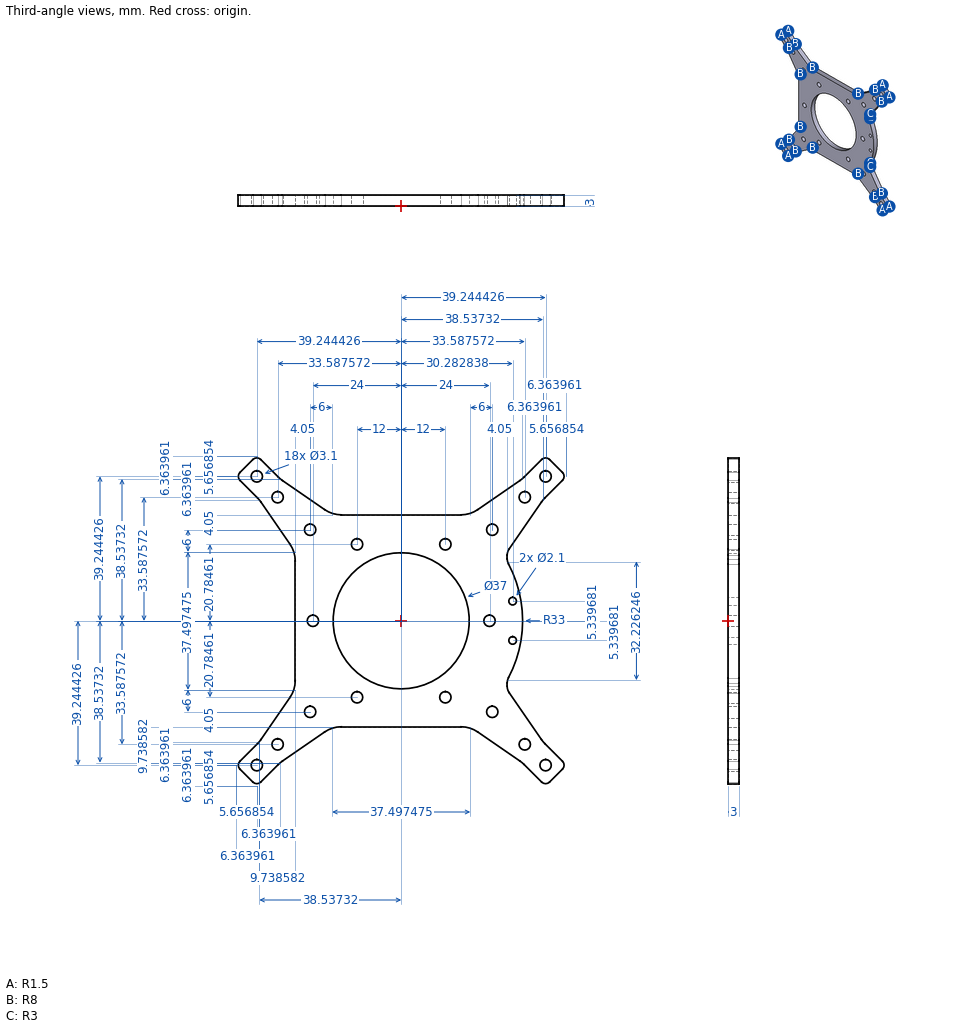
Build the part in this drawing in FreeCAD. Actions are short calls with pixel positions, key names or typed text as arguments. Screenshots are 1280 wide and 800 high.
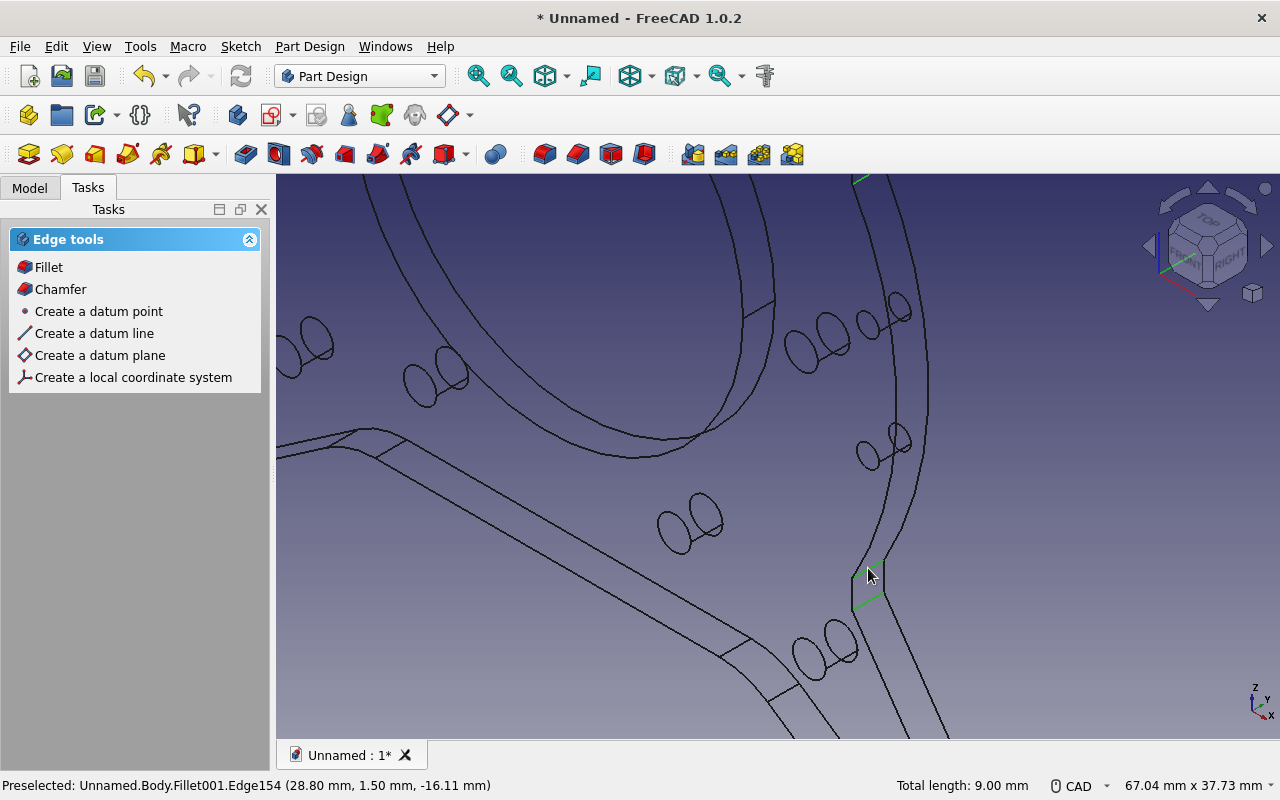
click(479, 76)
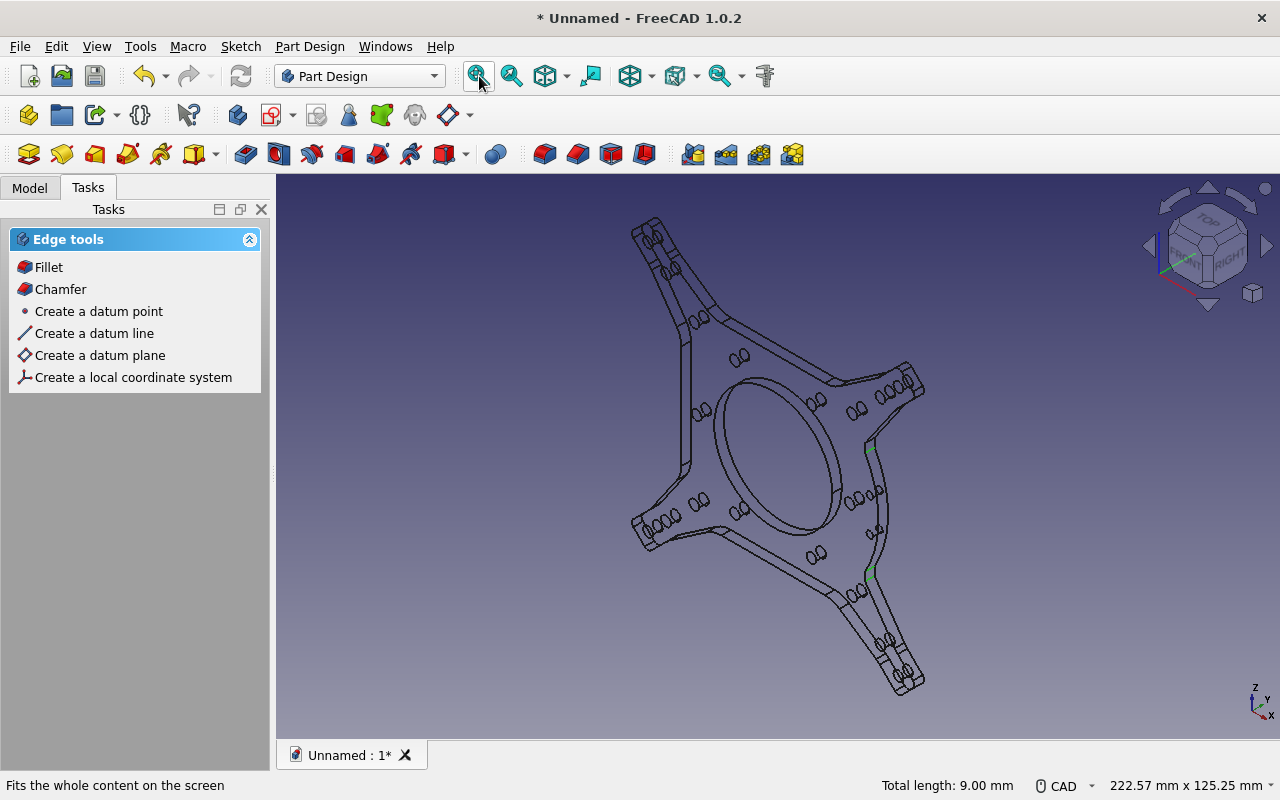
key(2)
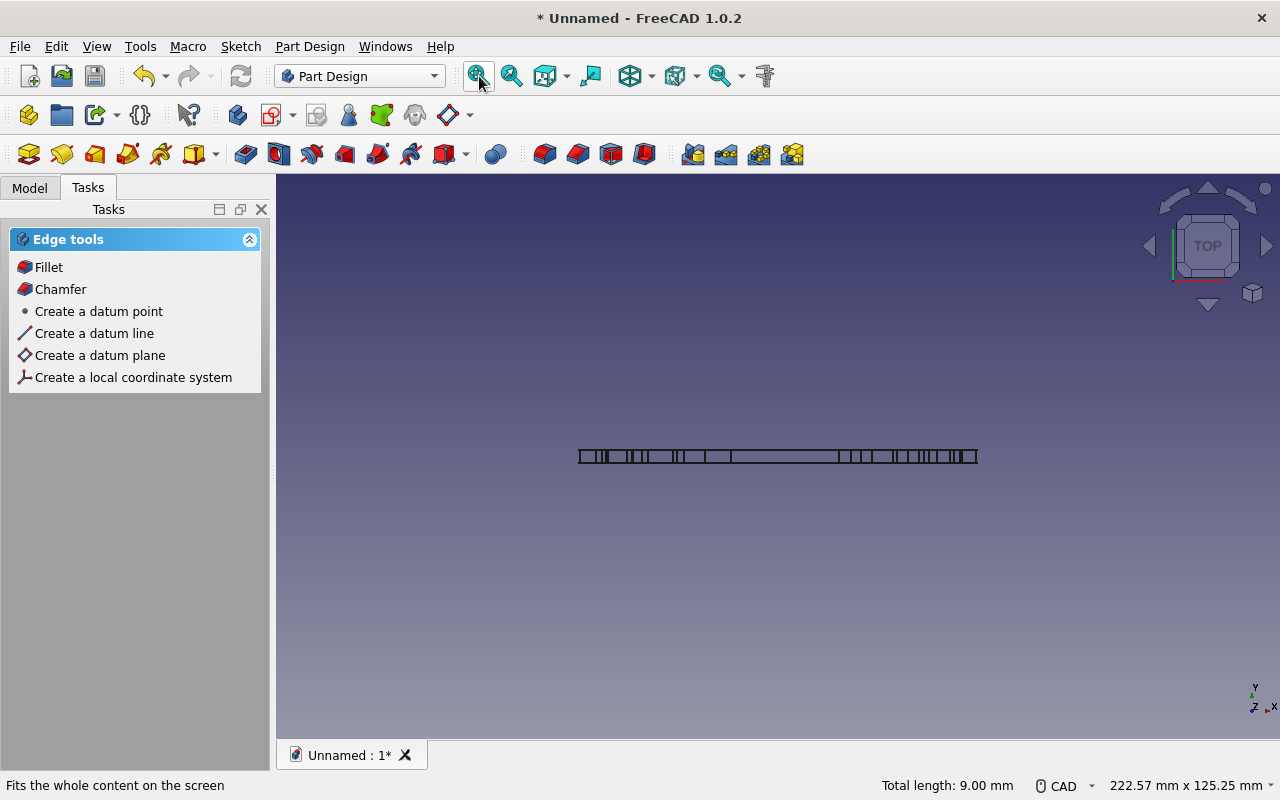
click(479, 76)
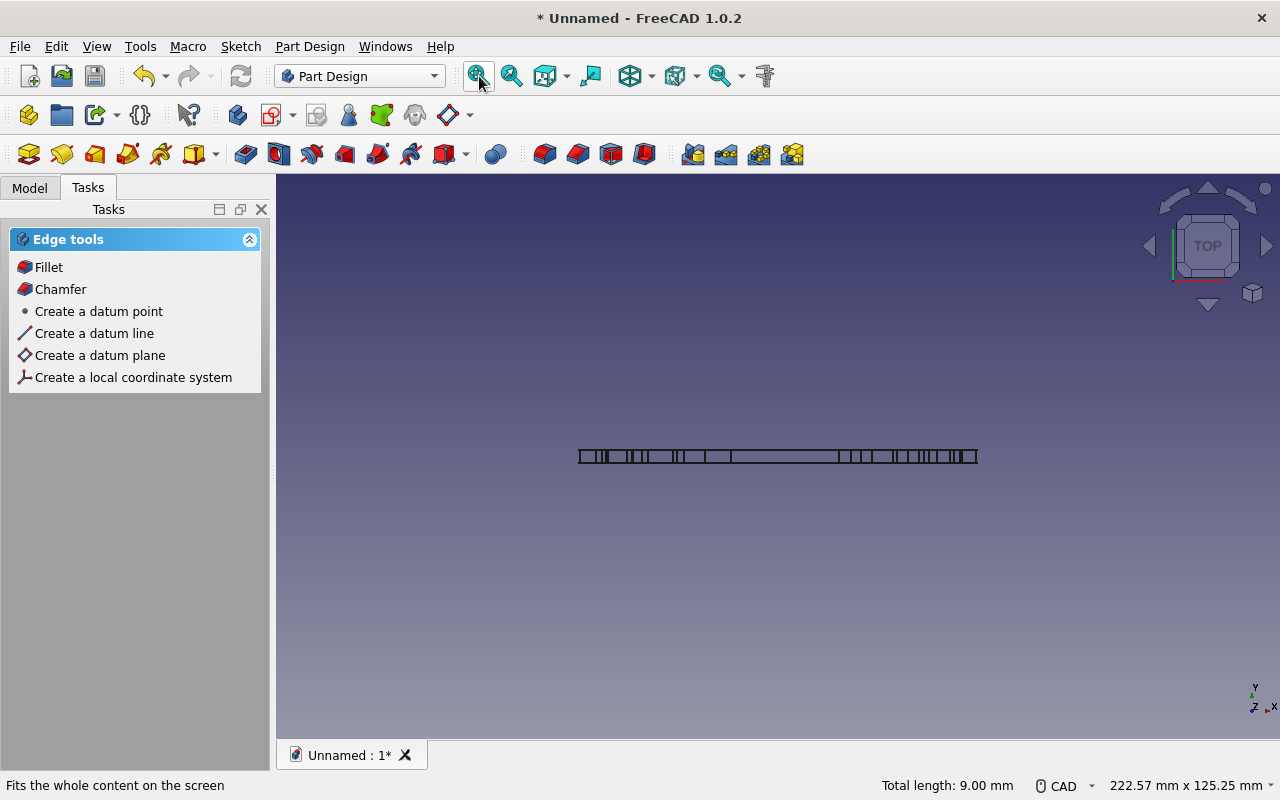
click(908, 455, ctrl)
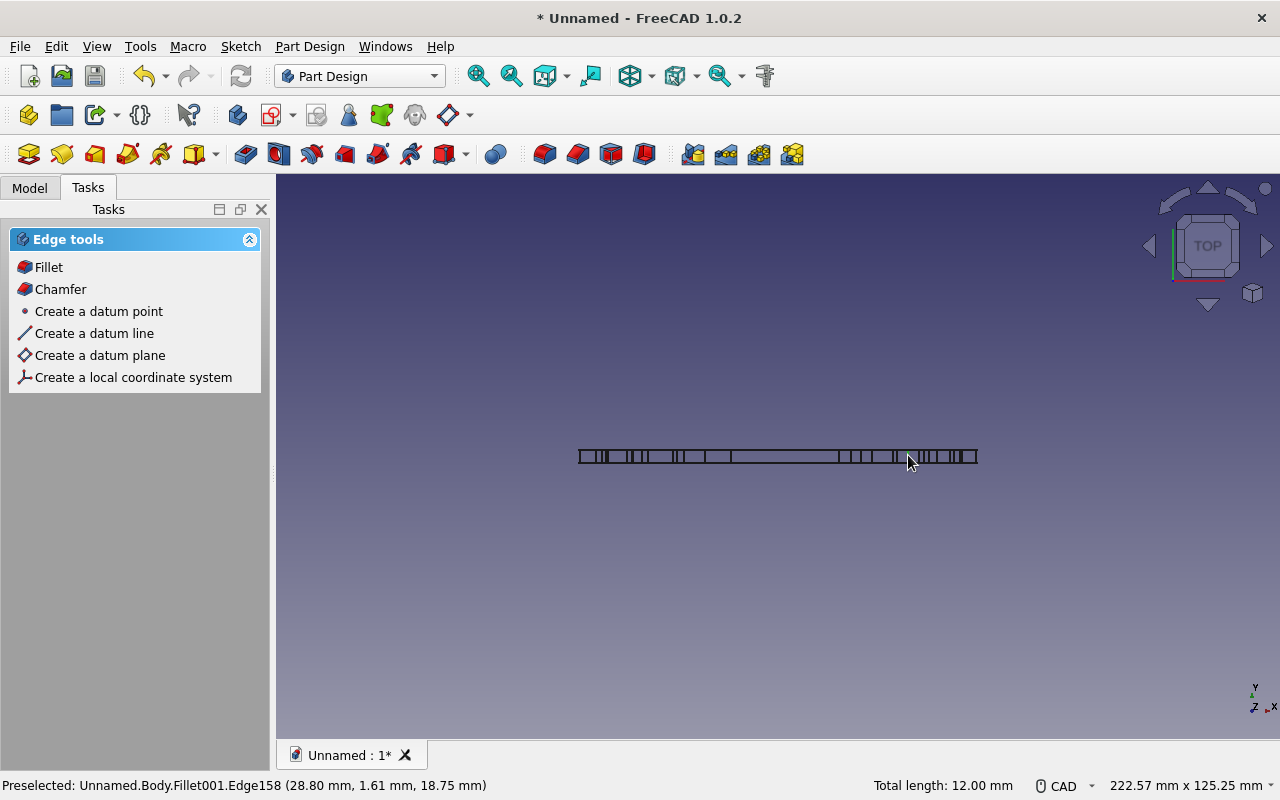
key(v)
key(1)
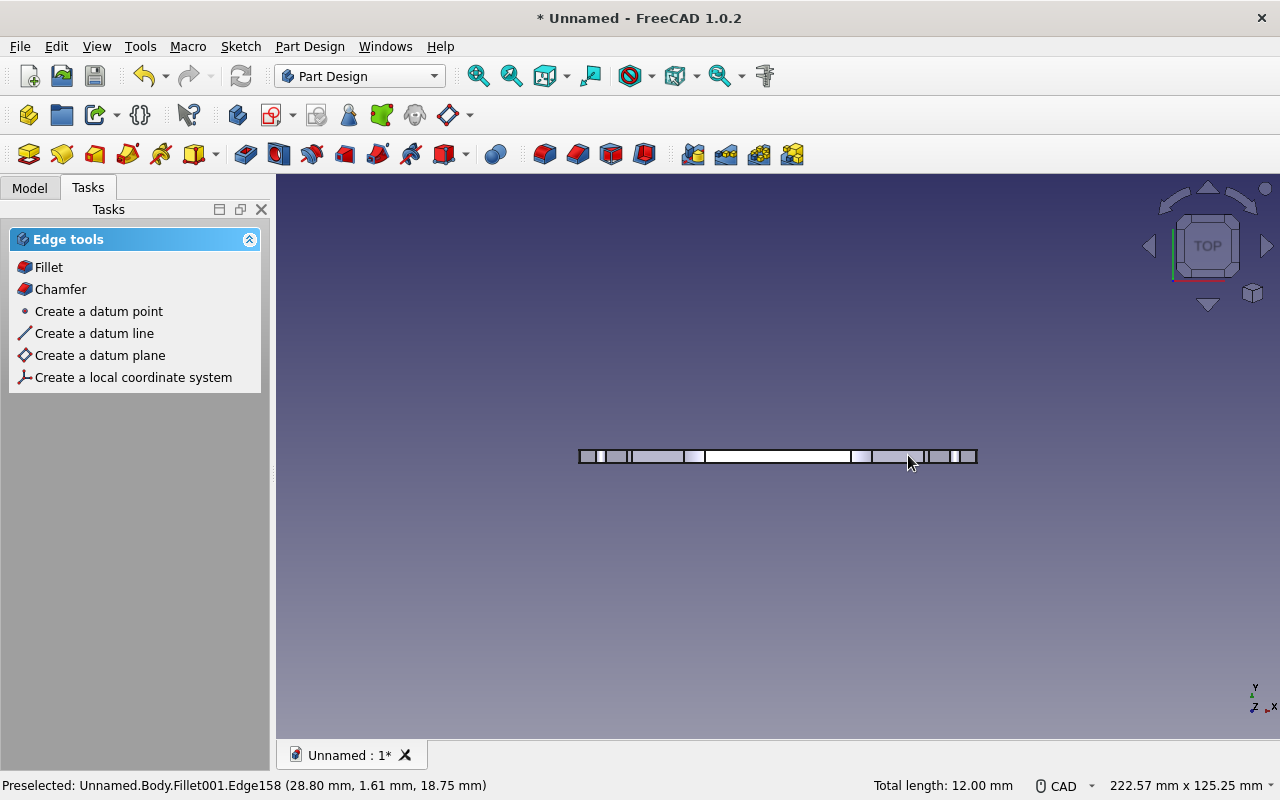
click(545, 154)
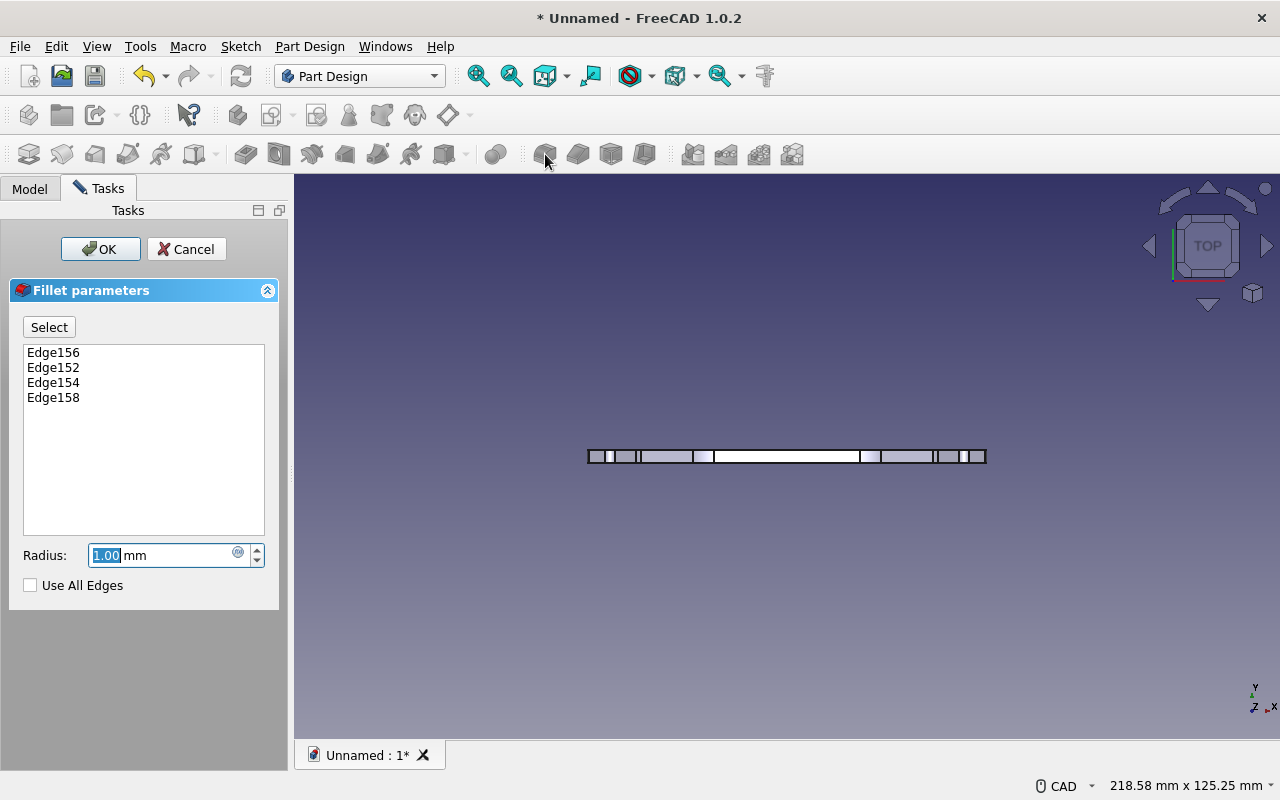
text(3)
key(Tab)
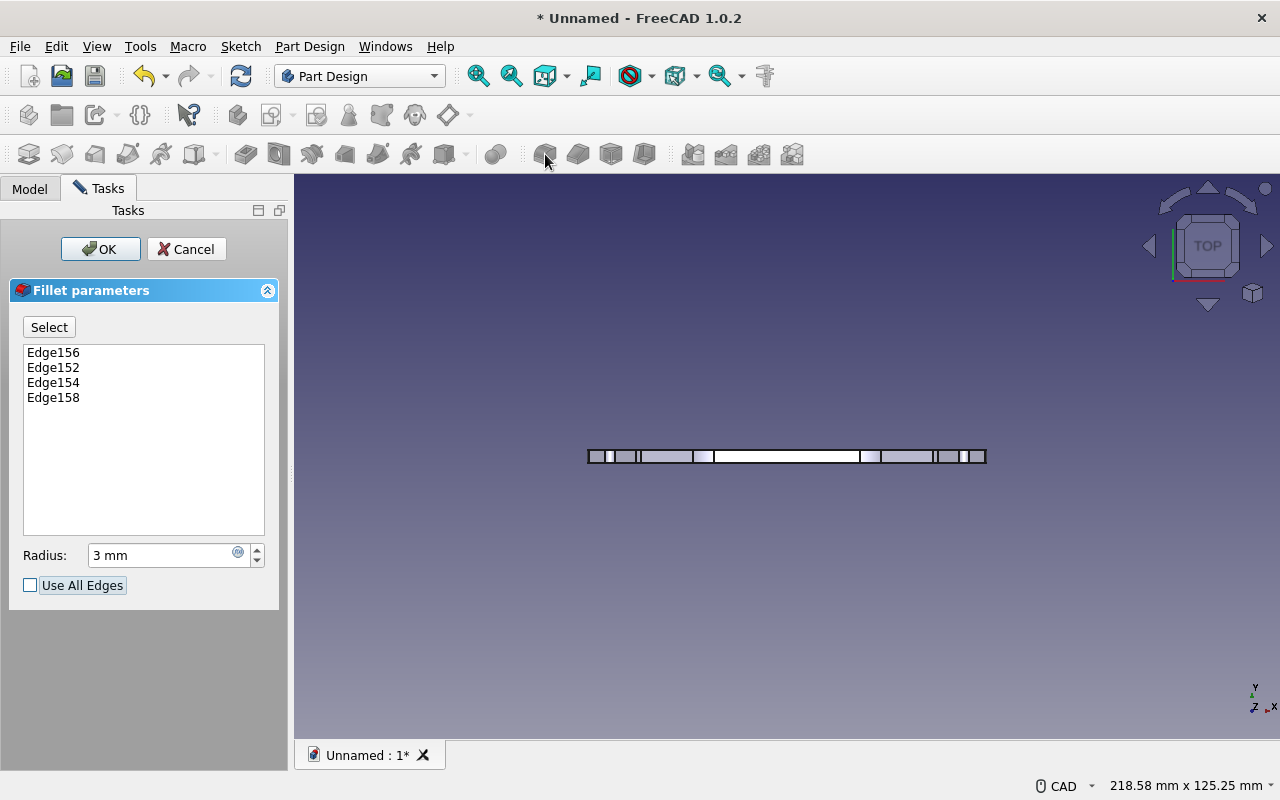
click(101, 249)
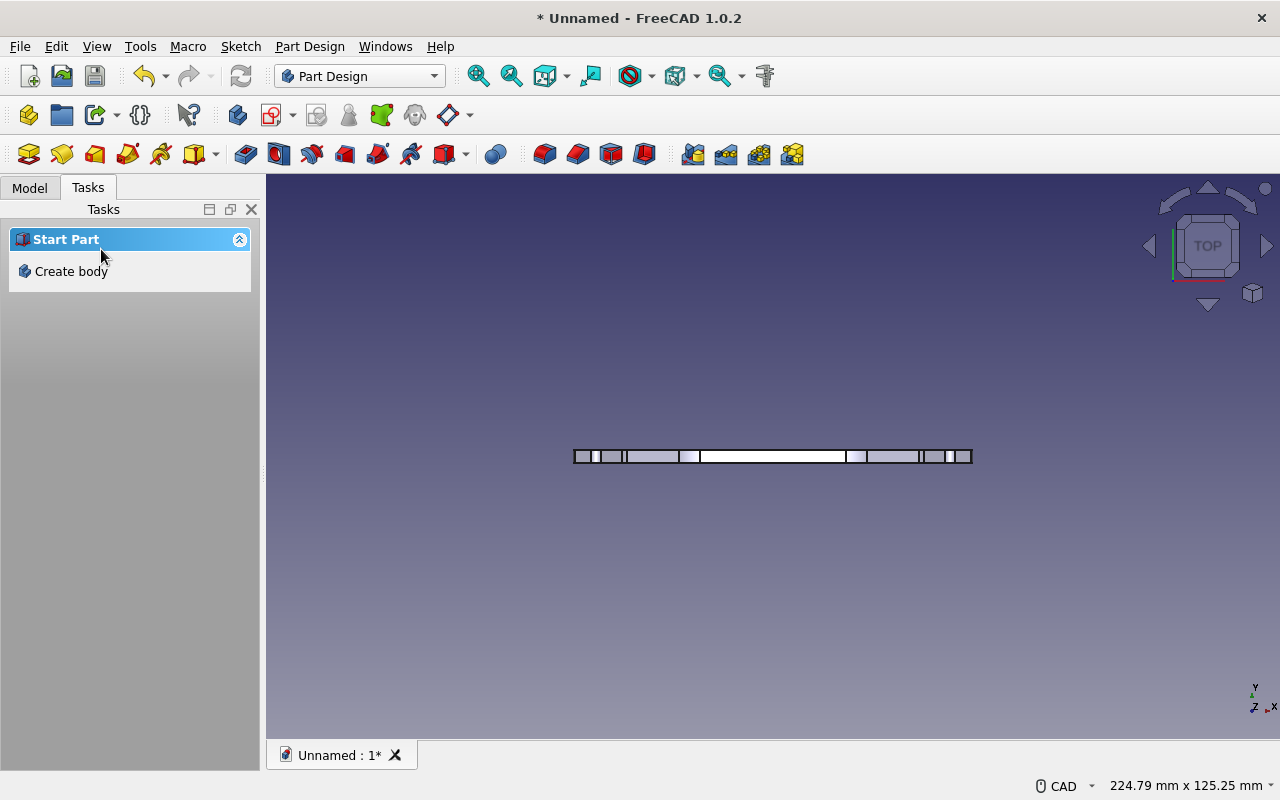
key(0)